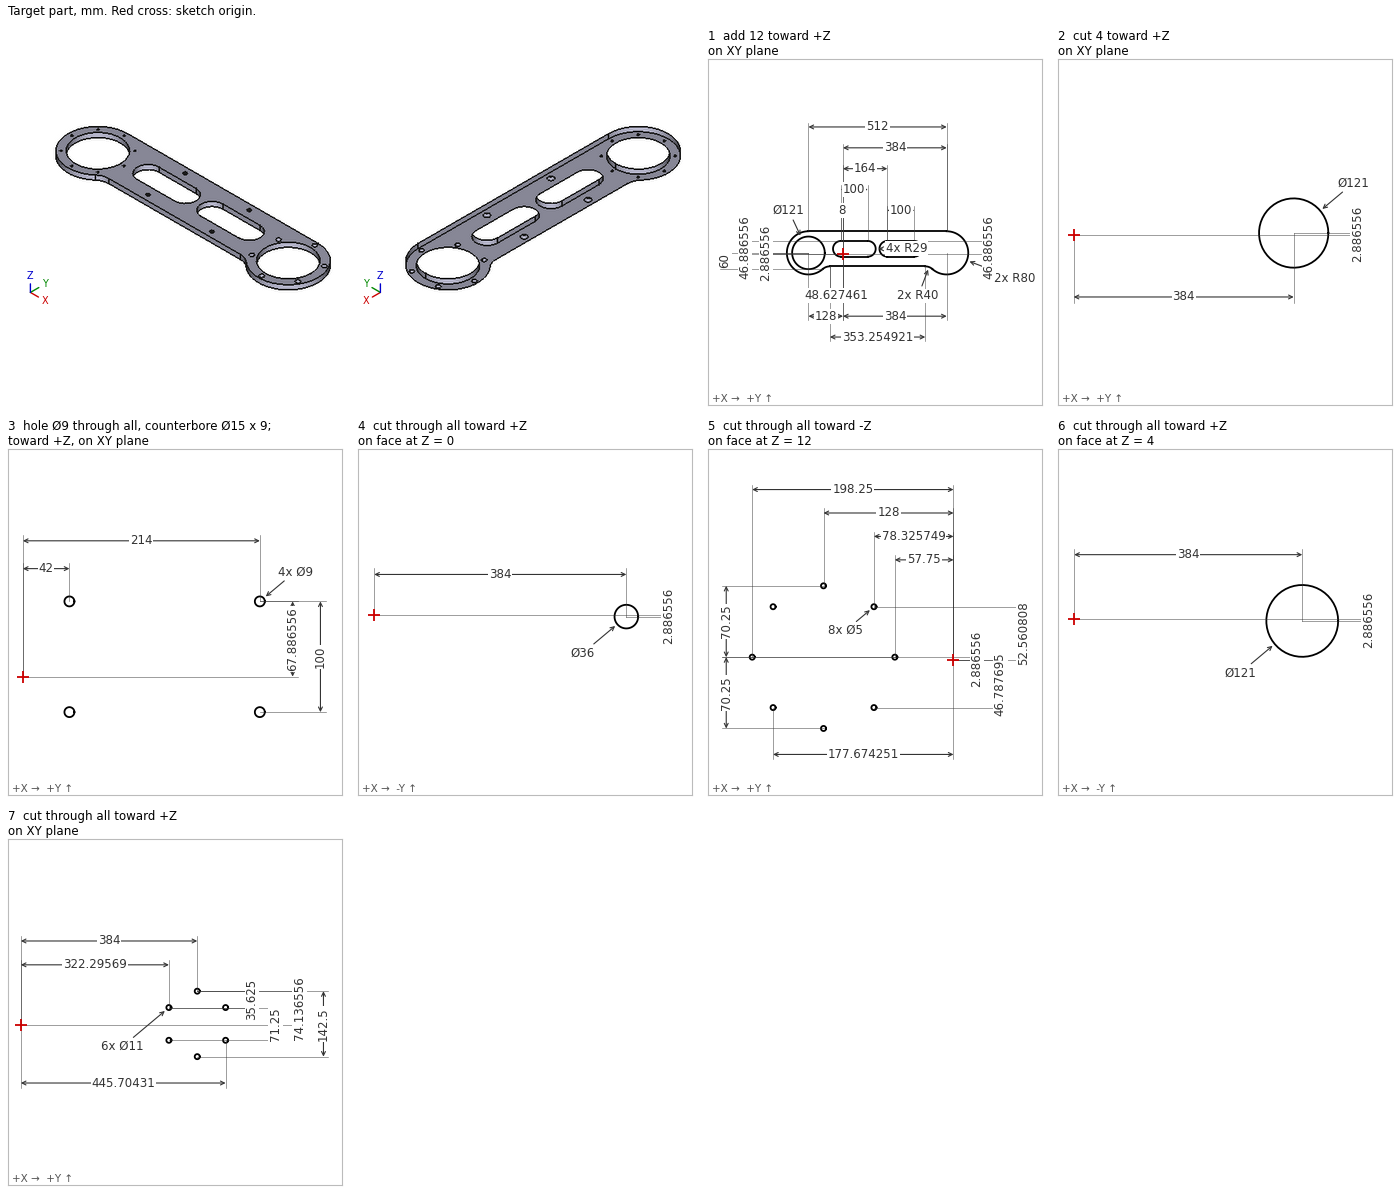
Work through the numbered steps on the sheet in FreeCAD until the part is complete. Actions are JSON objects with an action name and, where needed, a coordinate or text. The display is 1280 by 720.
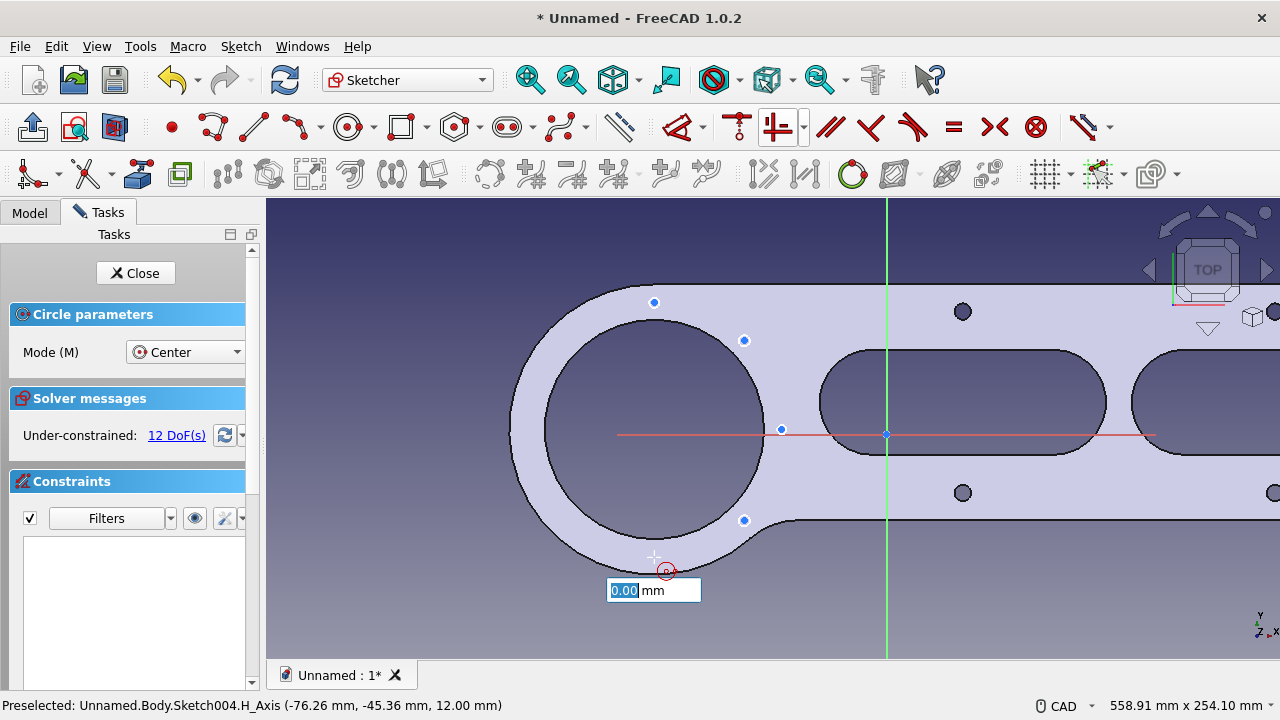
{"action": "scroll", "coordinate": [658, 554], "scroll_direction": "up", "scroll_amount": 7}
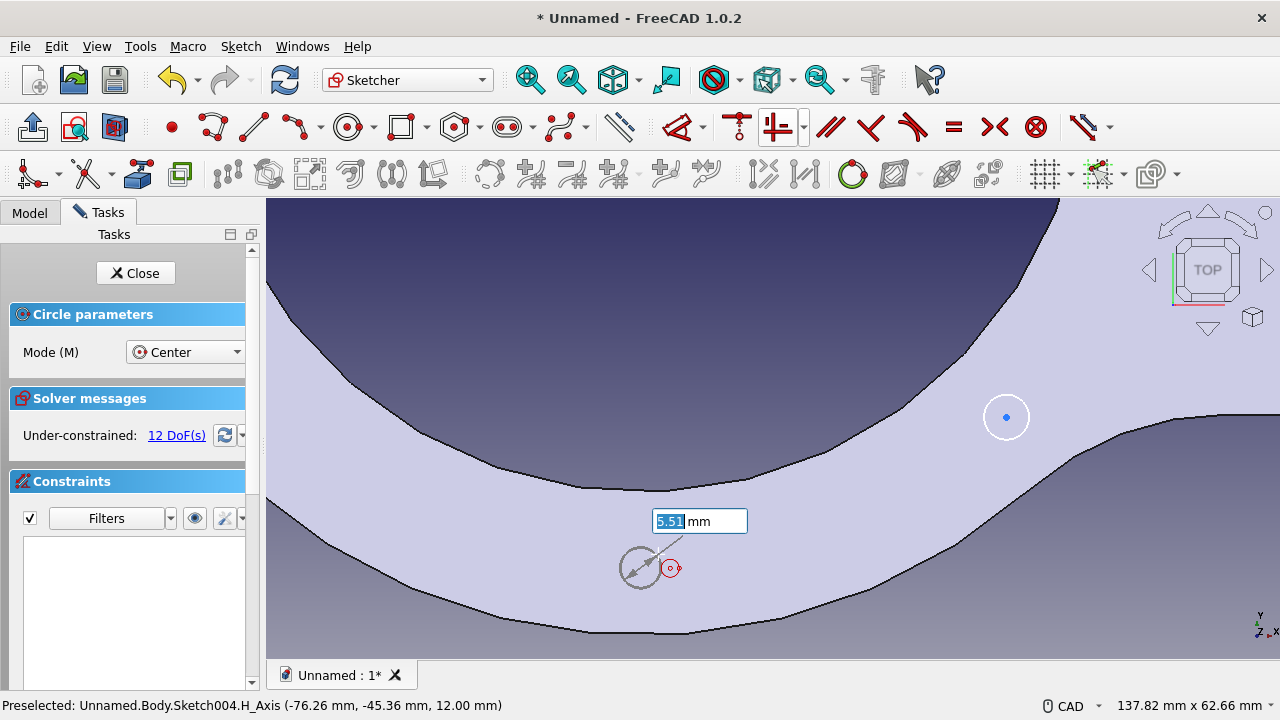
{"action": "left_click", "coordinate": [655, 551]}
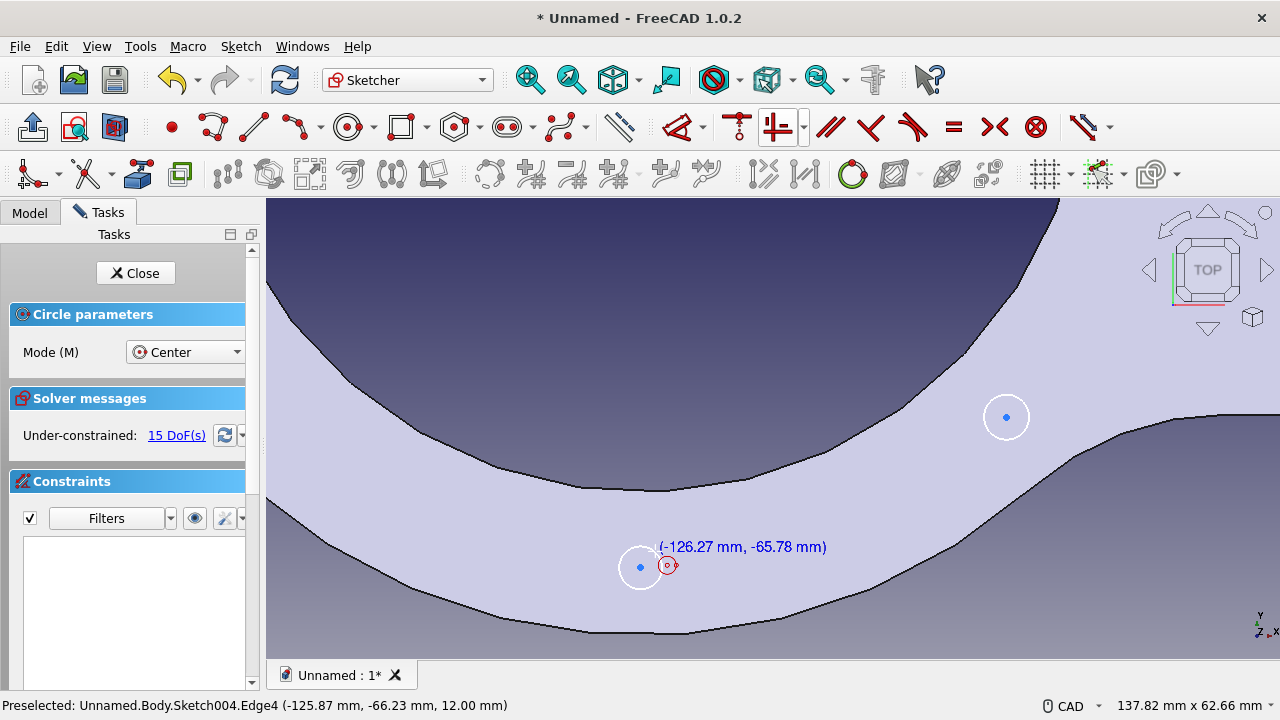
{"action": "scroll", "coordinate": [658, 553], "scroll_direction": "down", "scroll_amount": 7}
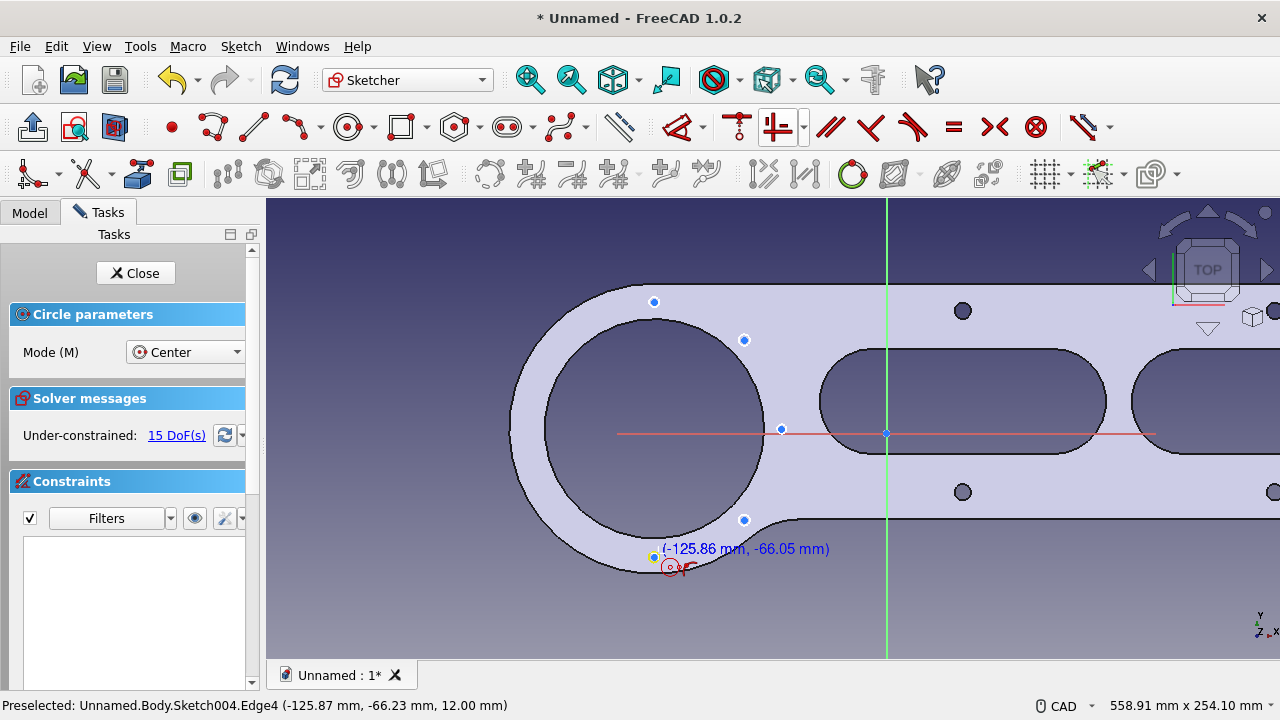
{"action": "scroll", "coordinate": [564, 519], "scroll_direction": "up", "scroll_amount": 9}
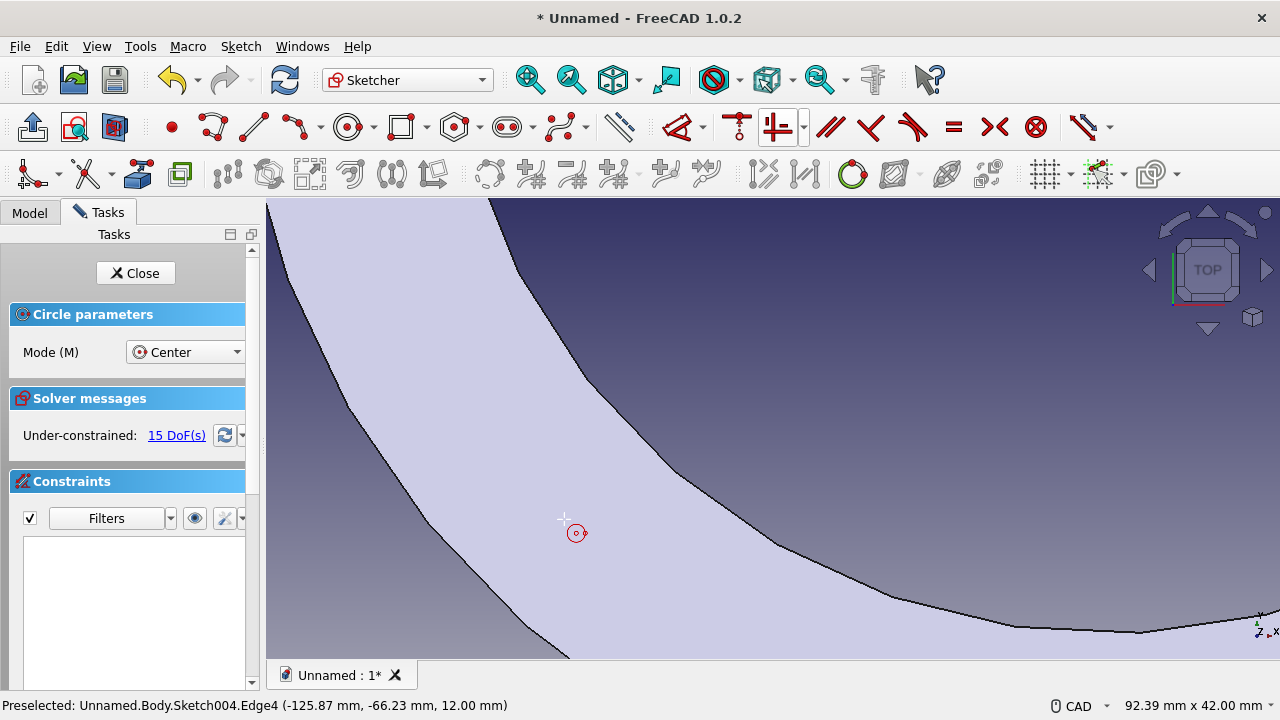
{"action": "scroll", "coordinate": [564, 519], "scroll_direction": "down", "scroll_amount": 9}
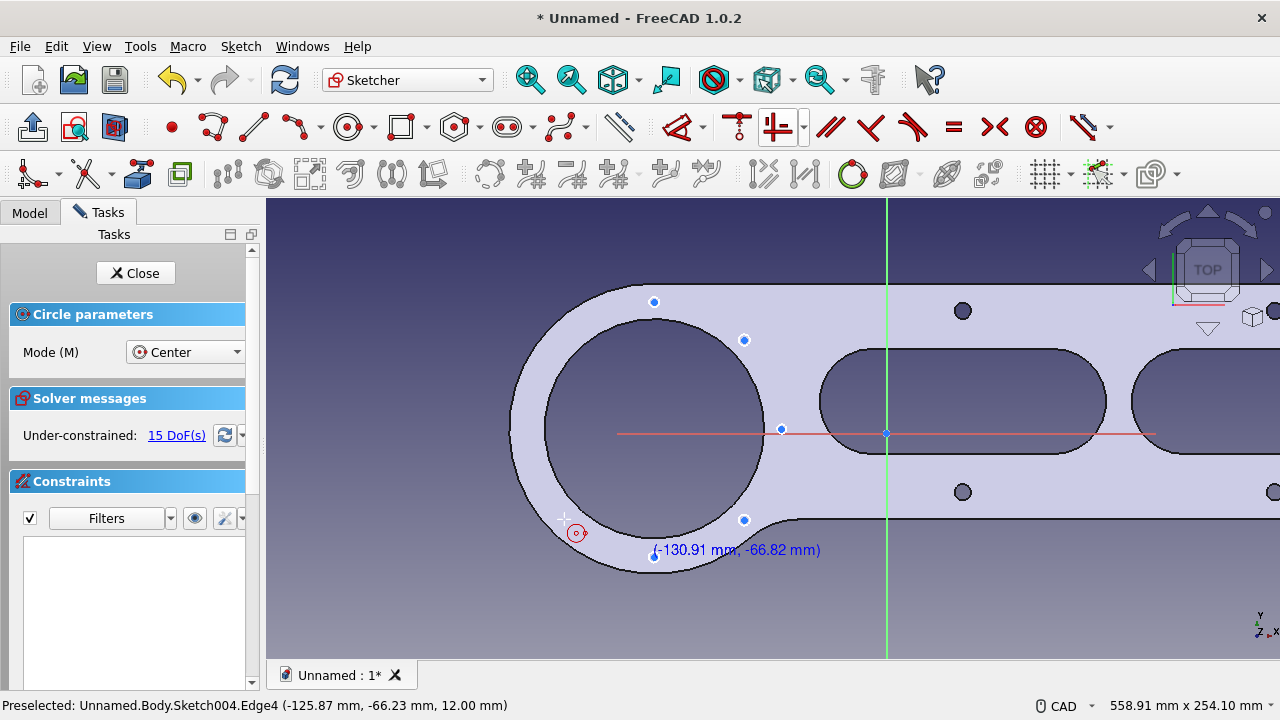
{"action": "left_click", "coordinate": [564, 519]}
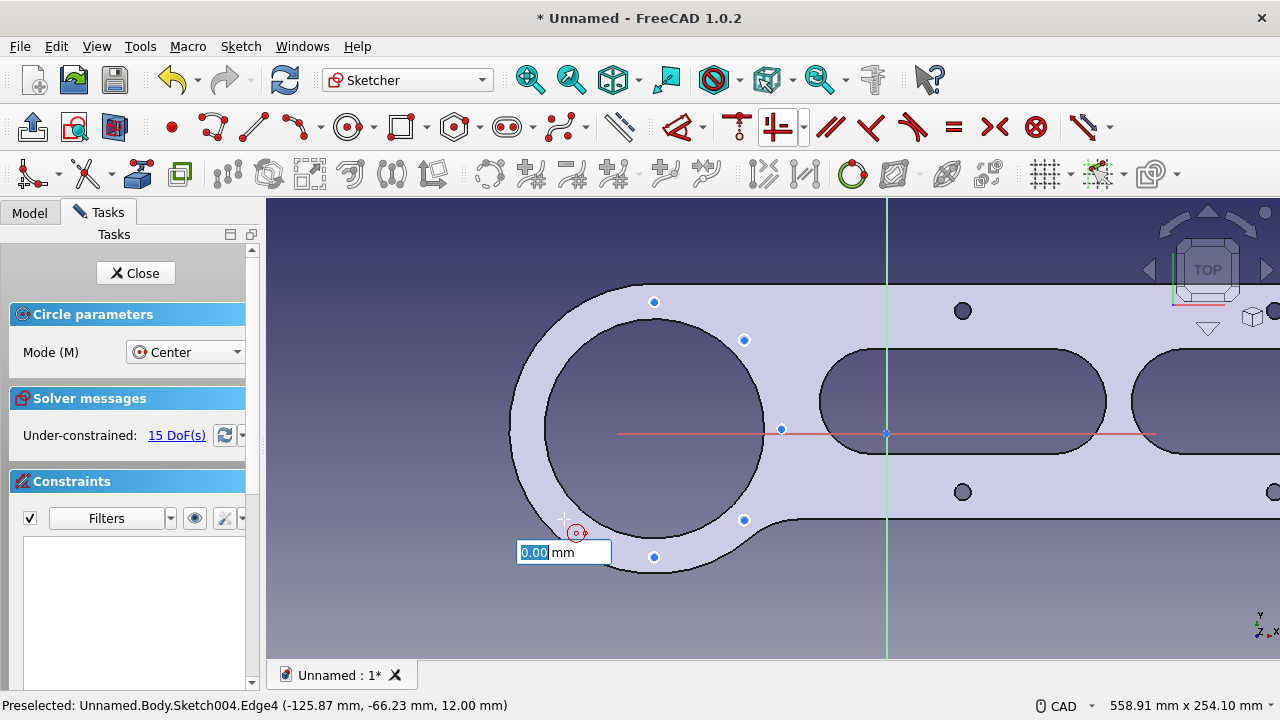
{"action": "scroll", "coordinate": [567, 516], "scroll_direction": "up", "scroll_amount": 7}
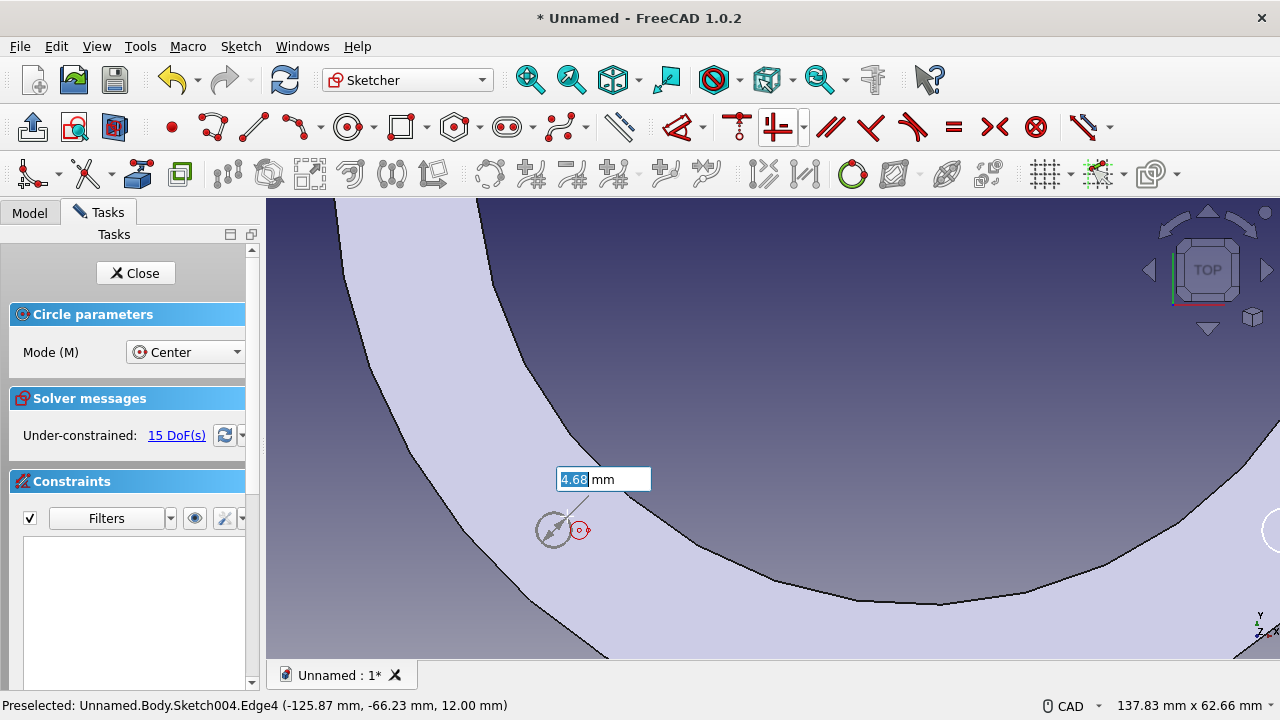
{"action": "left_click", "coordinate": [568, 513]}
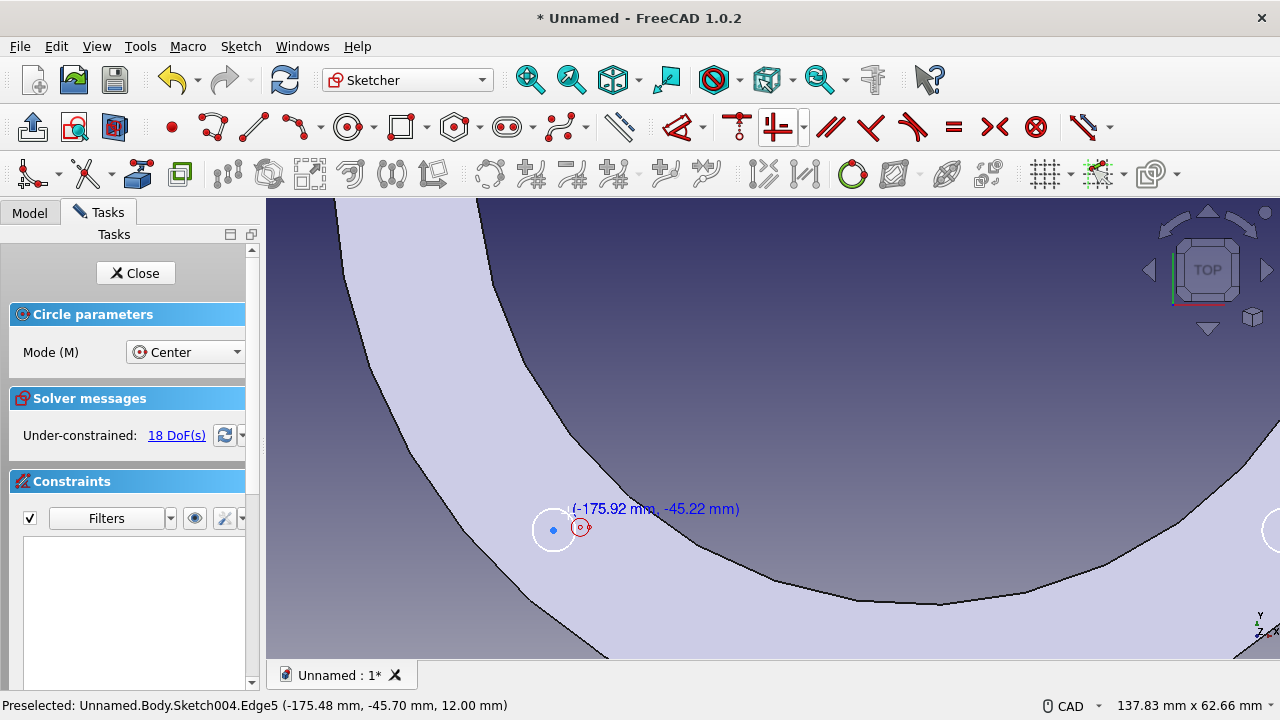
{"action": "scroll", "coordinate": [567, 516], "scroll_direction": "down", "scroll_amount": 7}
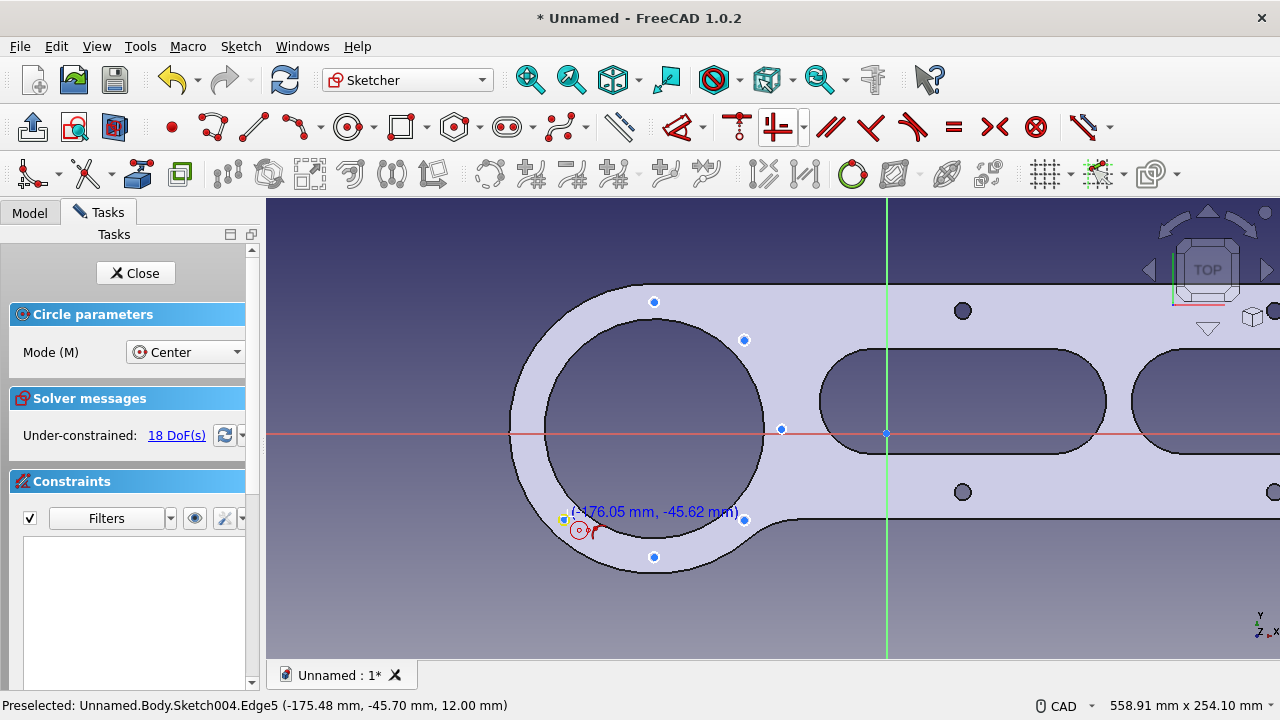
{"action": "scroll", "coordinate": [527, 429], "scroll_direction": "up", "scroll_amount": 9}